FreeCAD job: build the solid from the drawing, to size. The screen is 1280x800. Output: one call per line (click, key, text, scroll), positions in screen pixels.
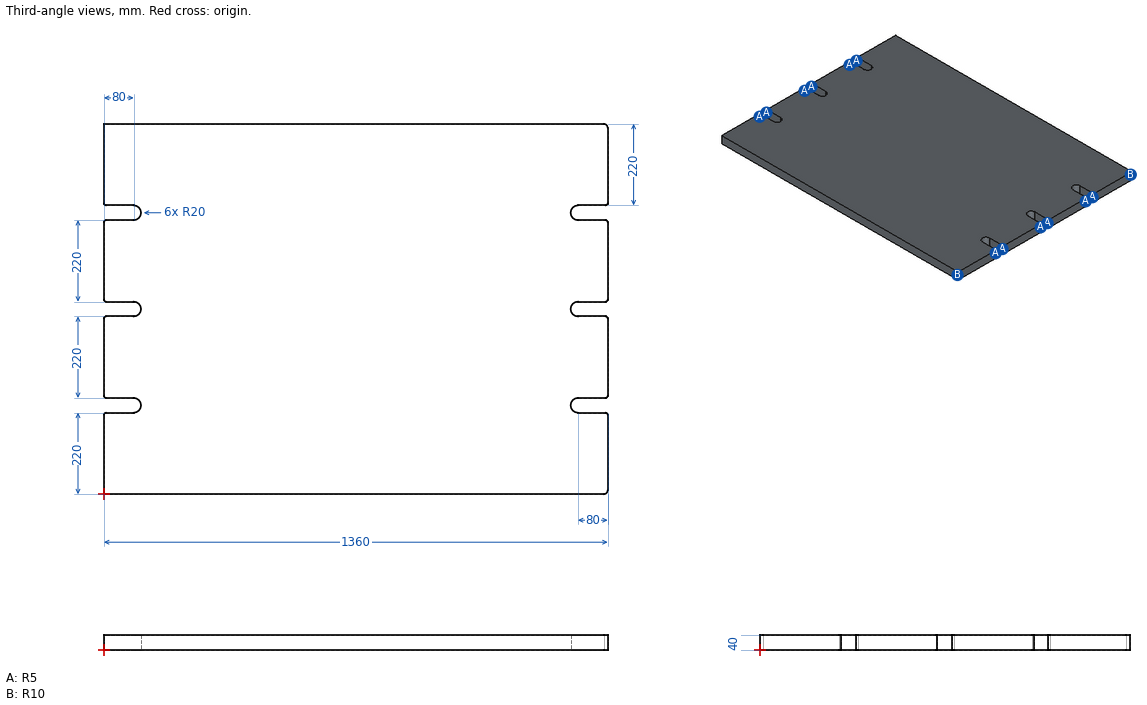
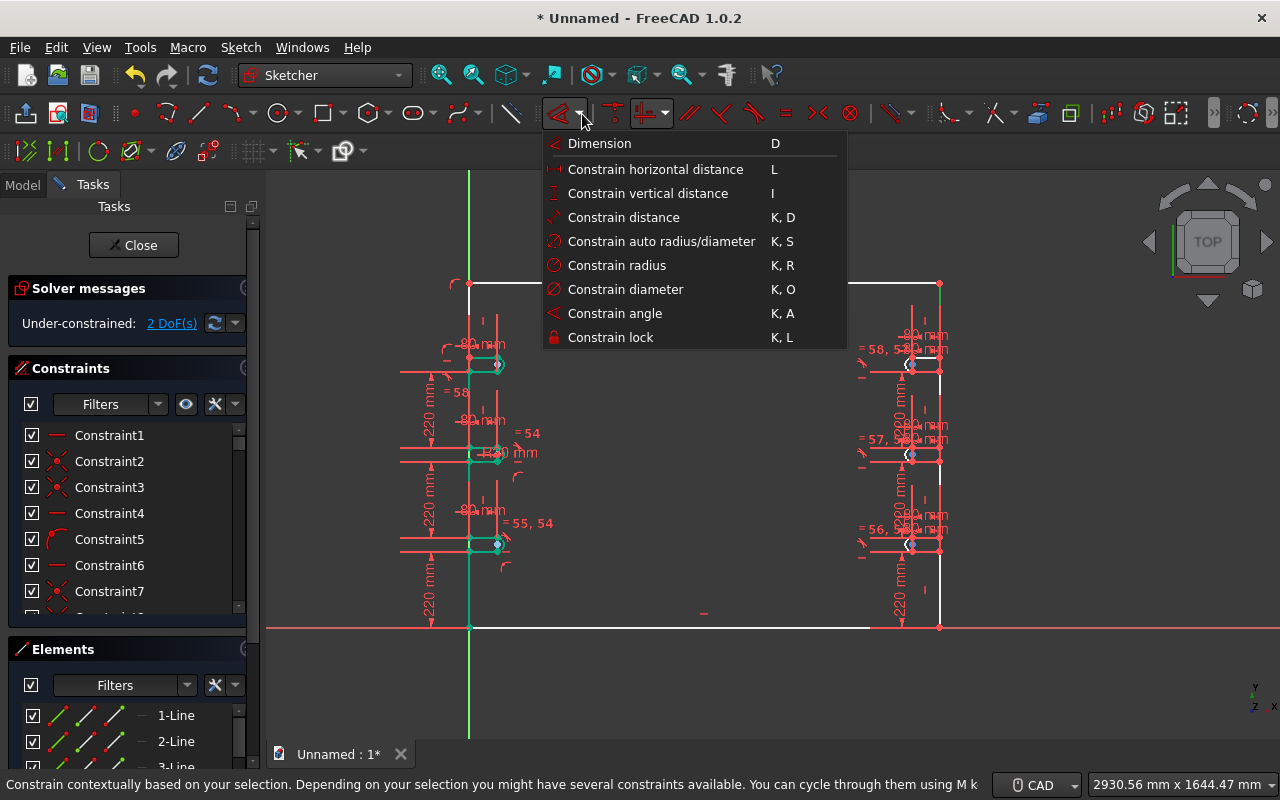
click(695, 193)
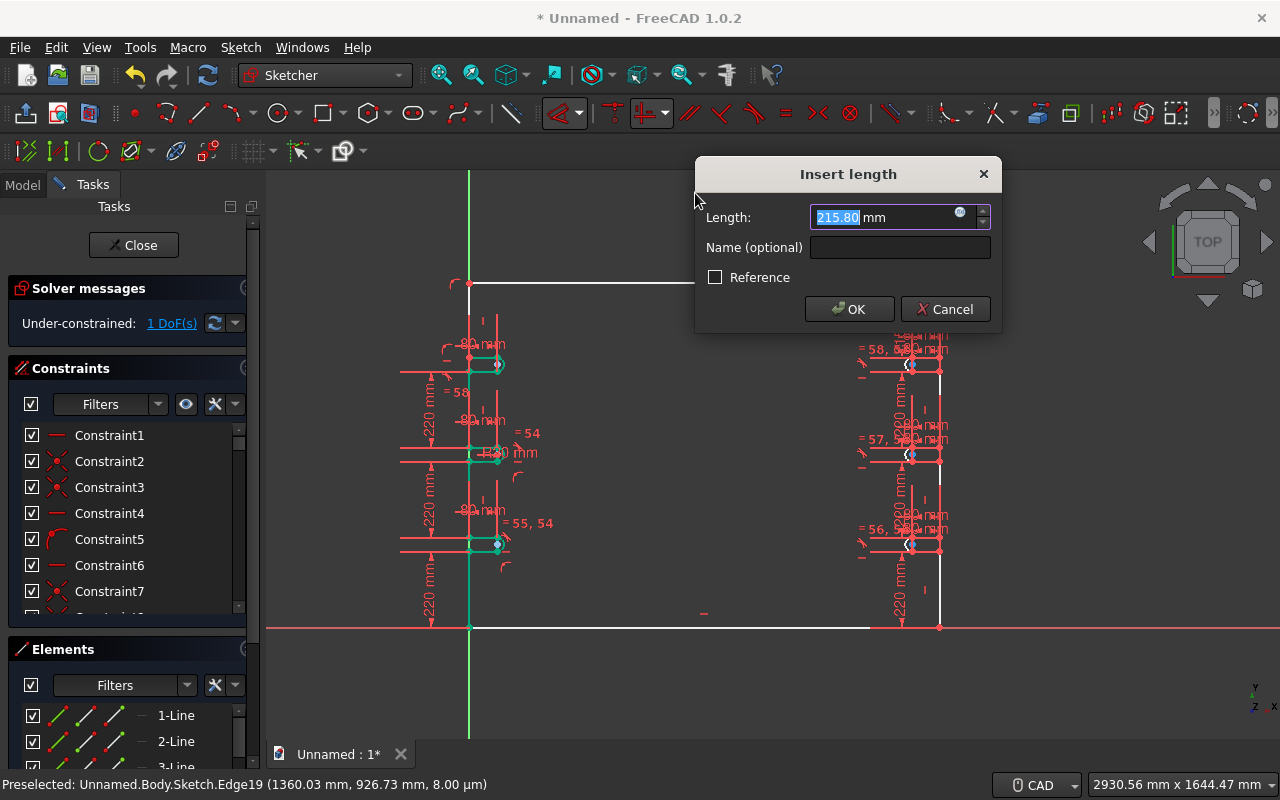
text(220)
key(Return)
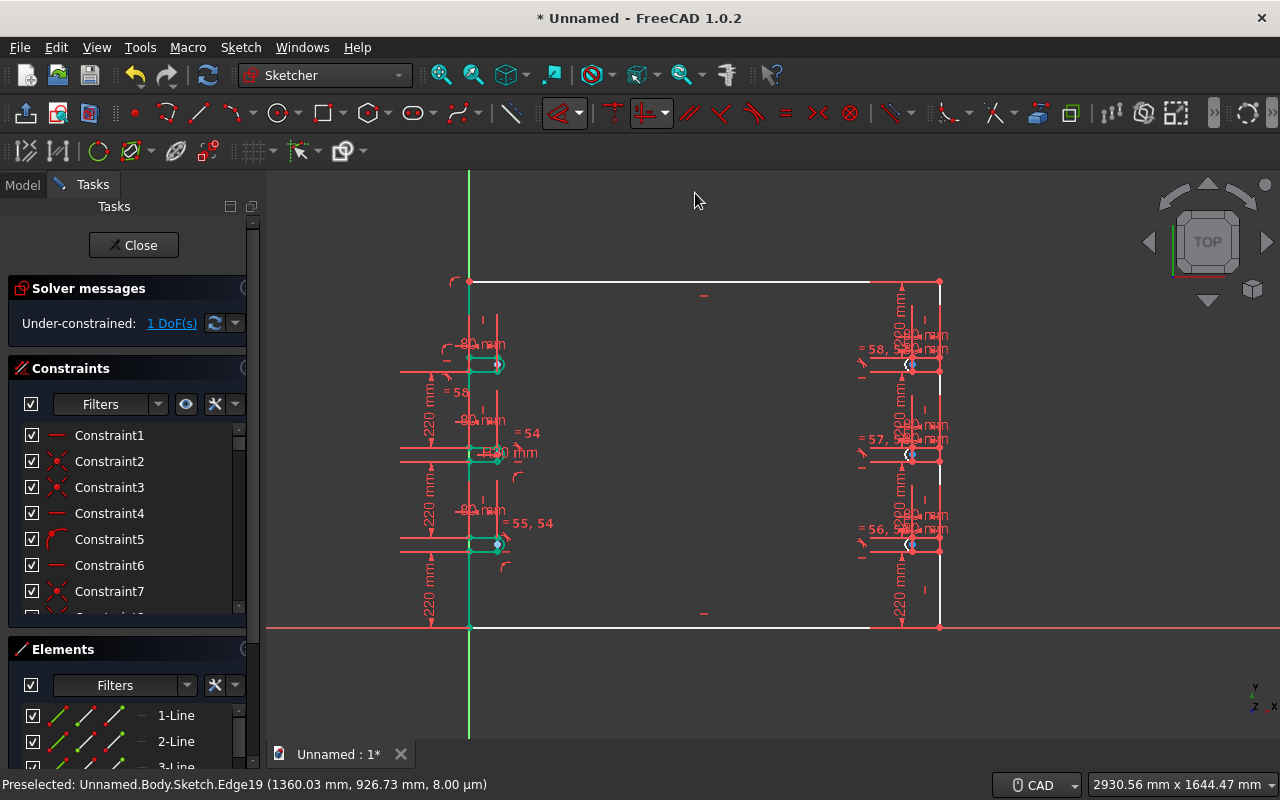
click(611, 628)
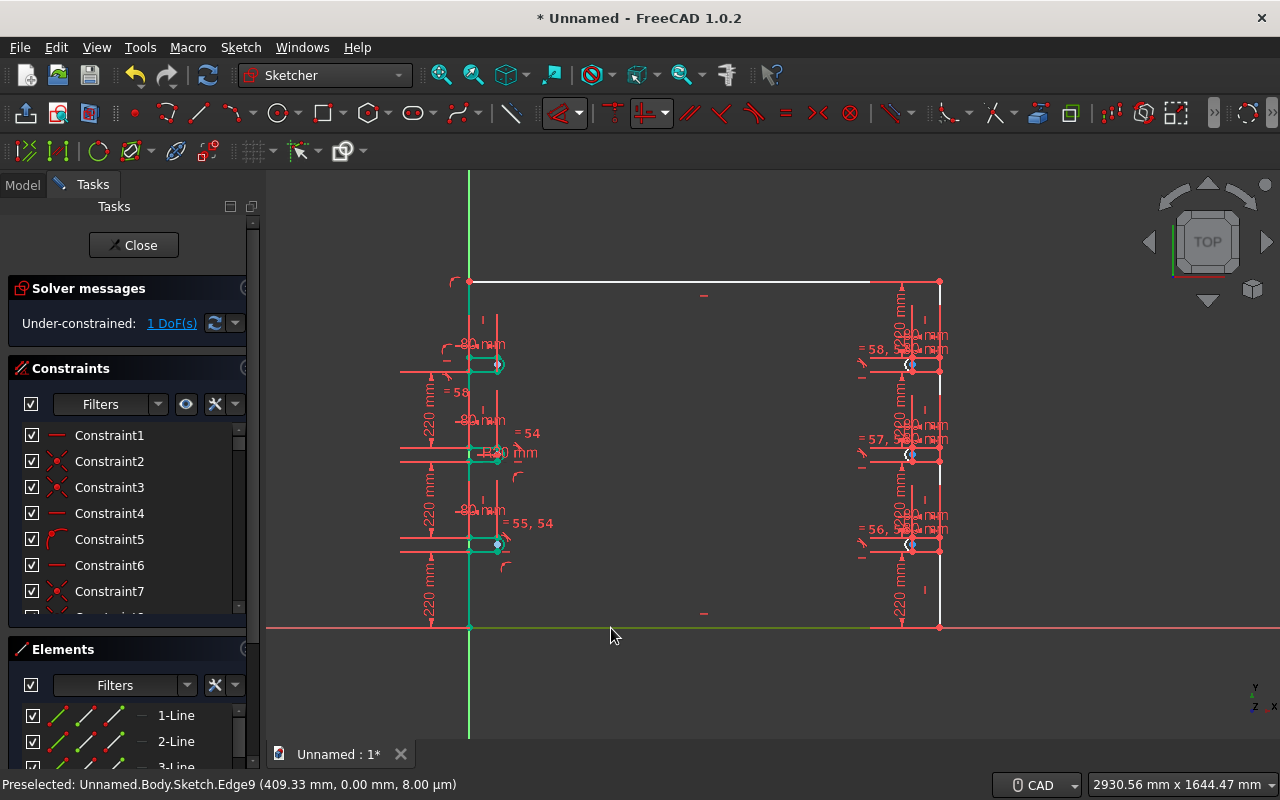
click(582, 114)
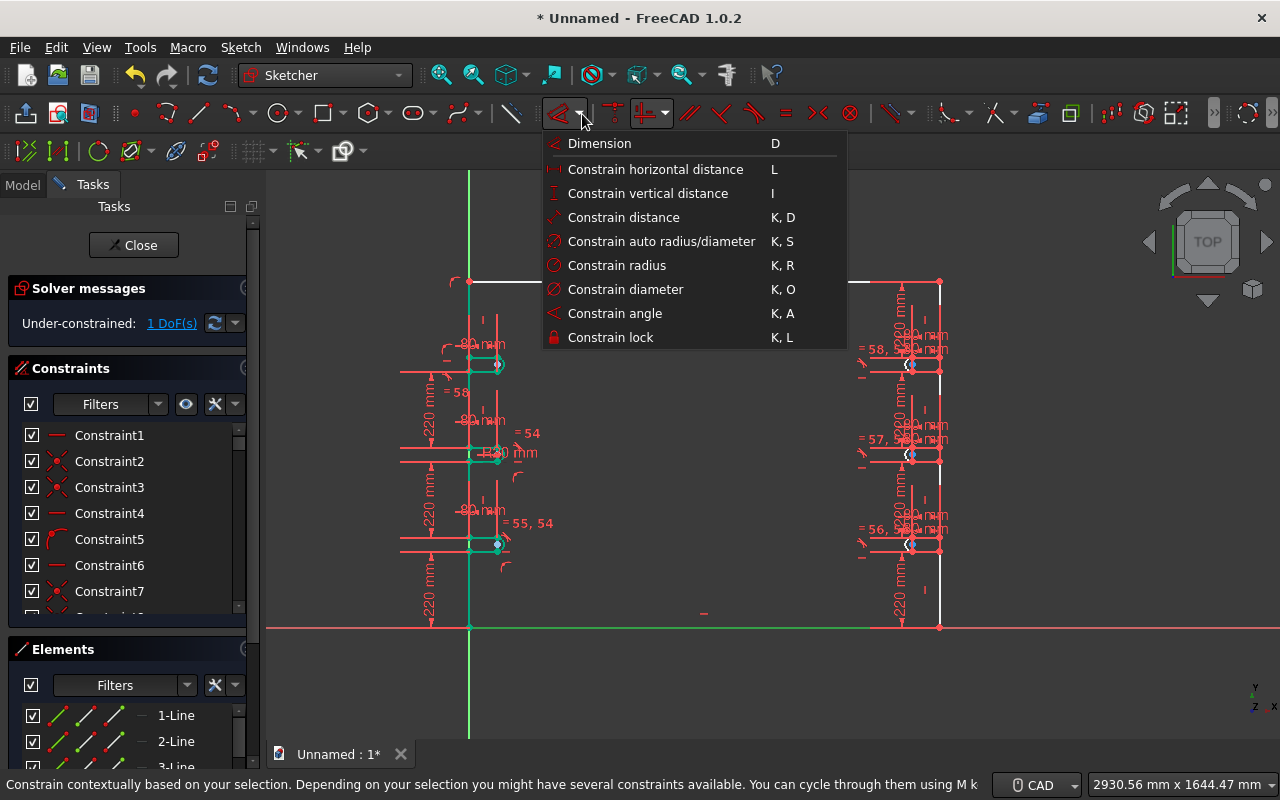
click(695, 169)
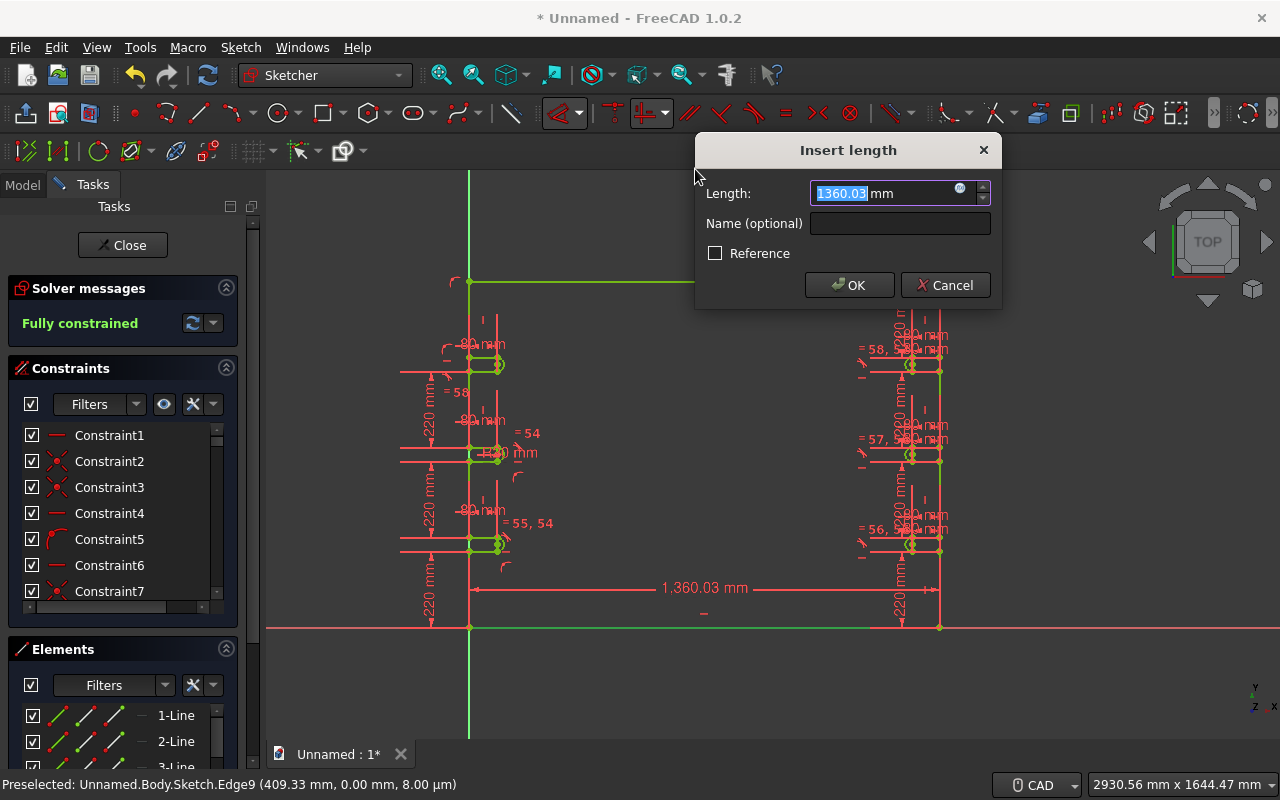
text(1360)
key(Return)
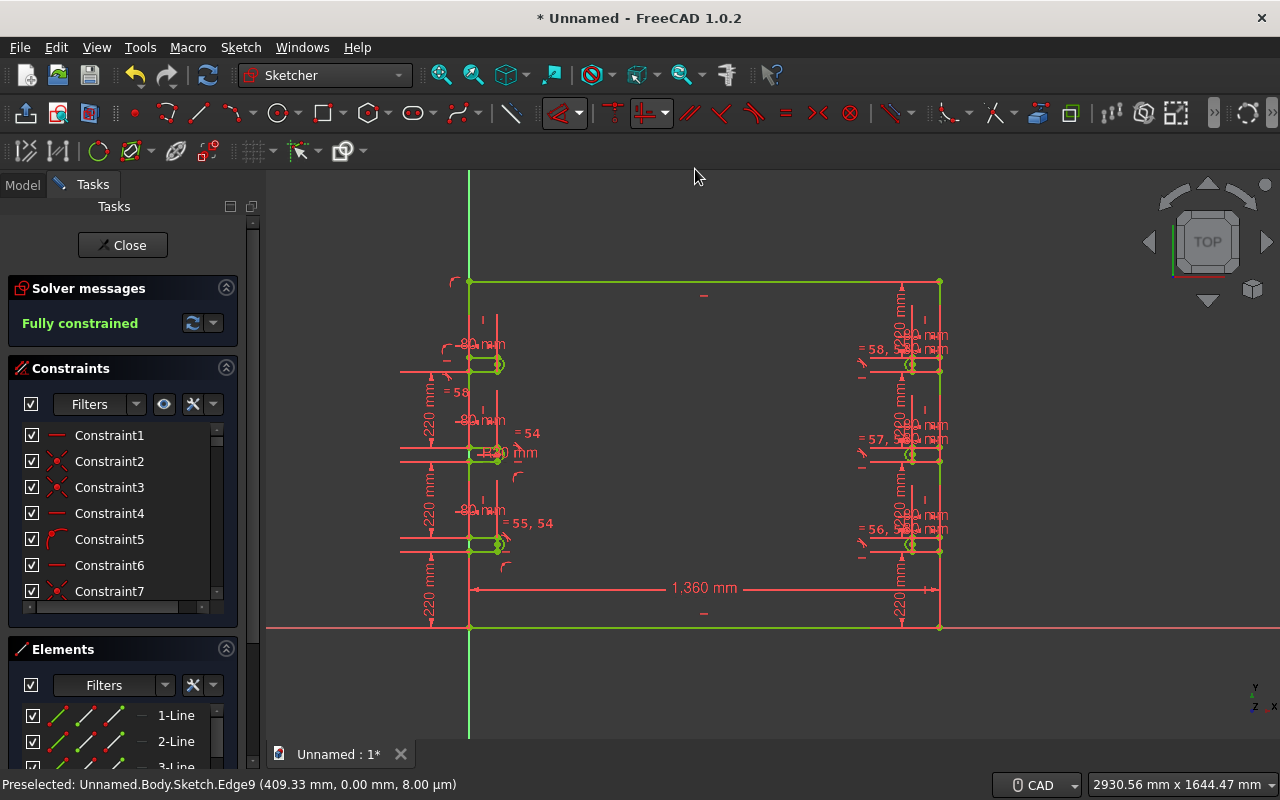
click(123, 245)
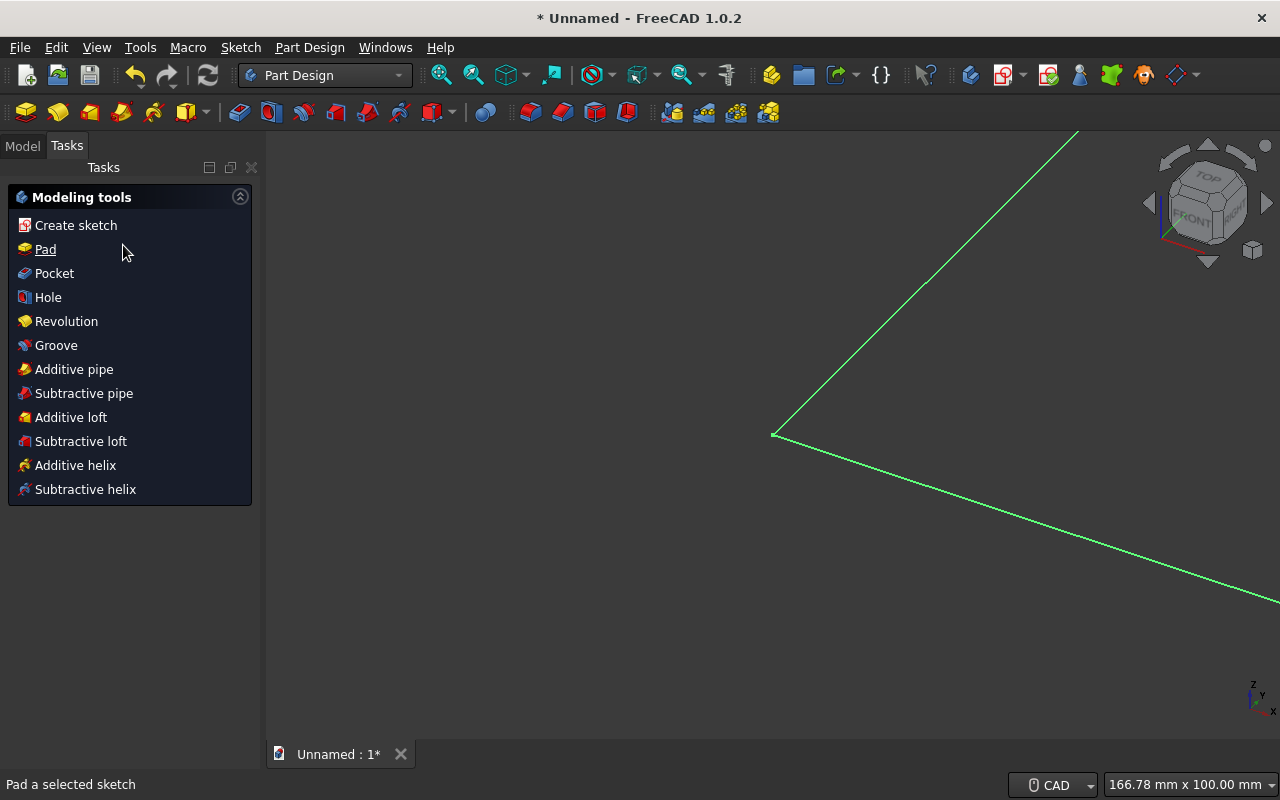
click(26, 112)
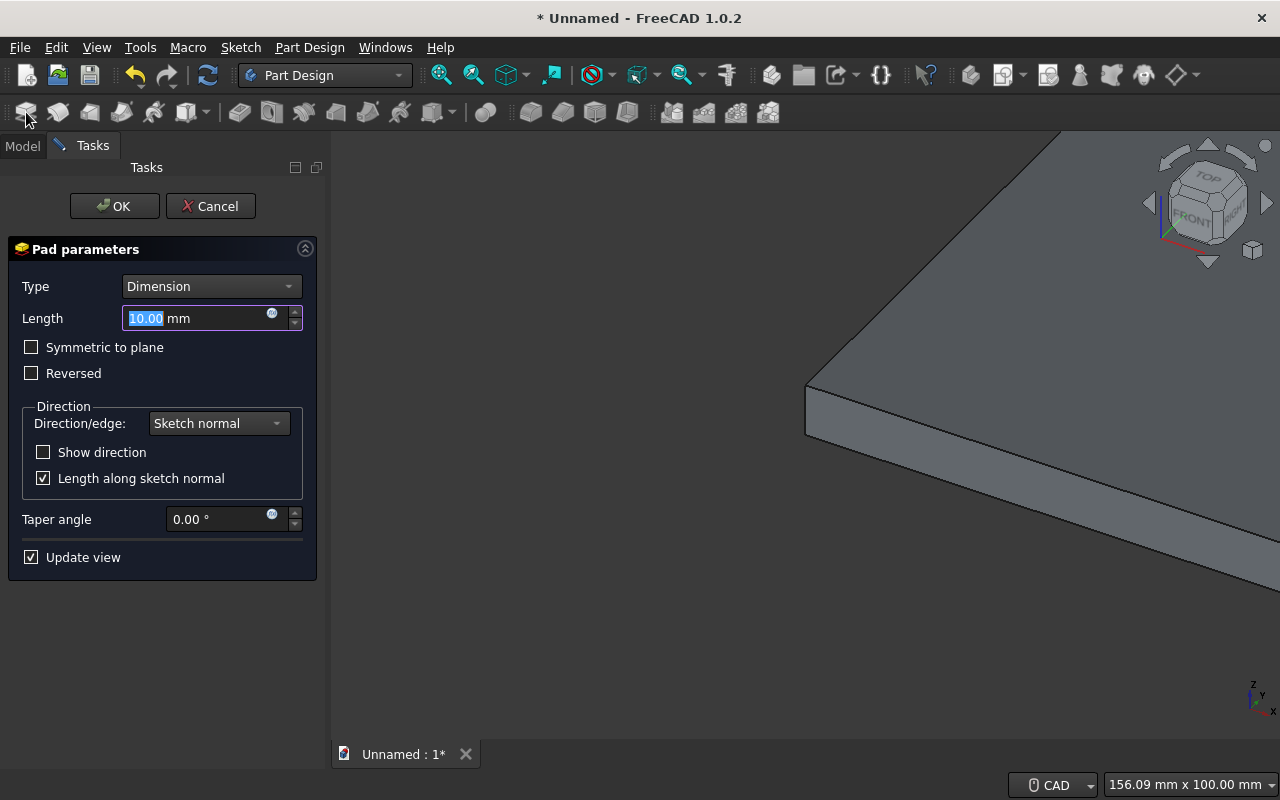
text(40)
key(Tab)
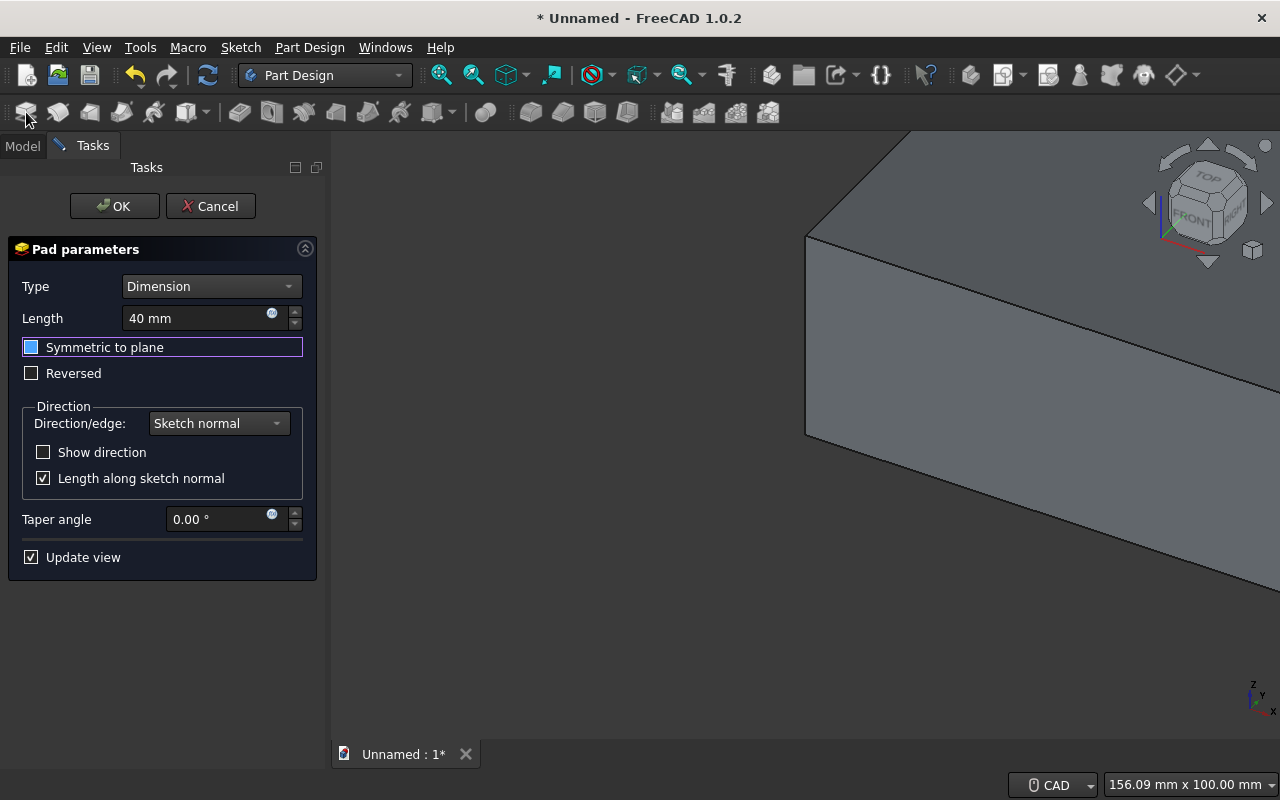
click(115, 206)